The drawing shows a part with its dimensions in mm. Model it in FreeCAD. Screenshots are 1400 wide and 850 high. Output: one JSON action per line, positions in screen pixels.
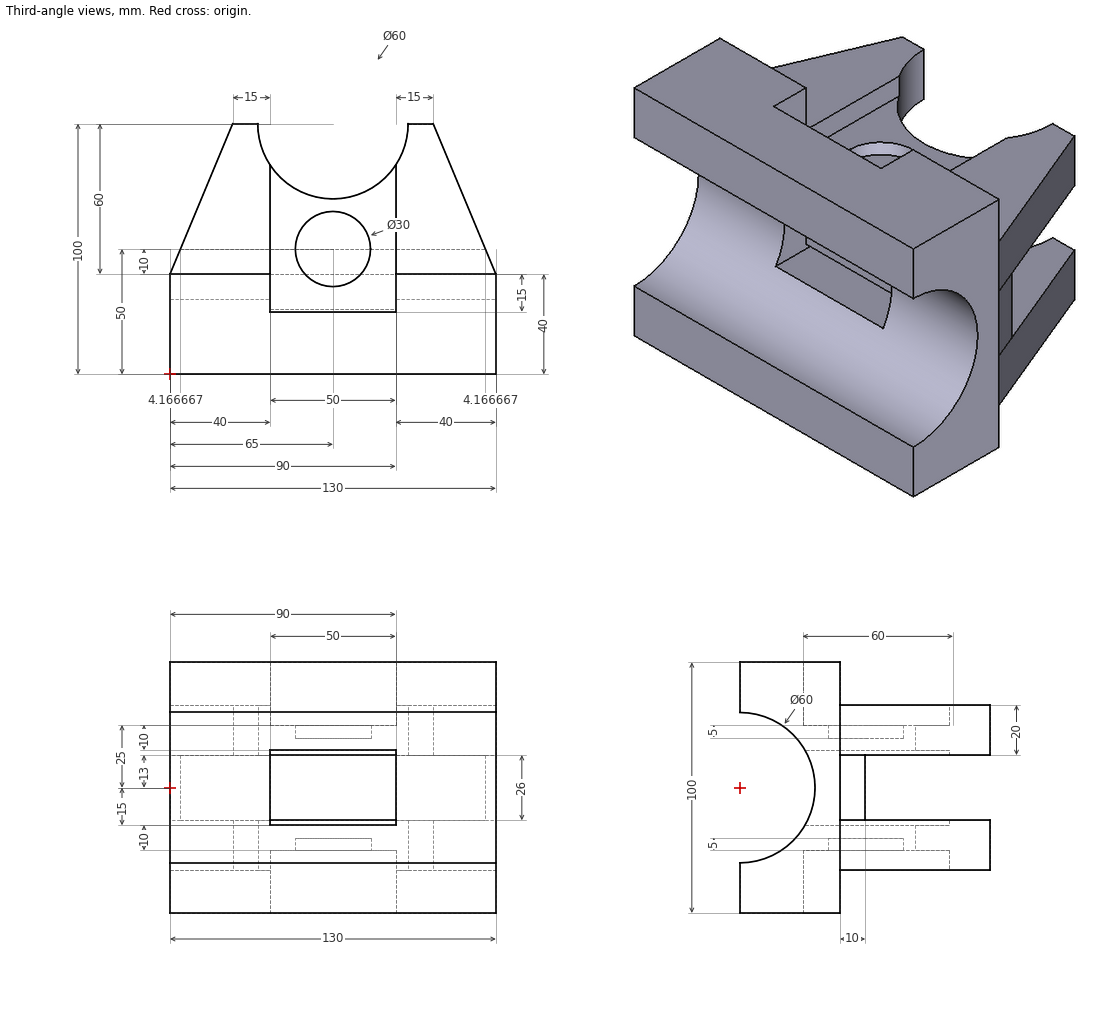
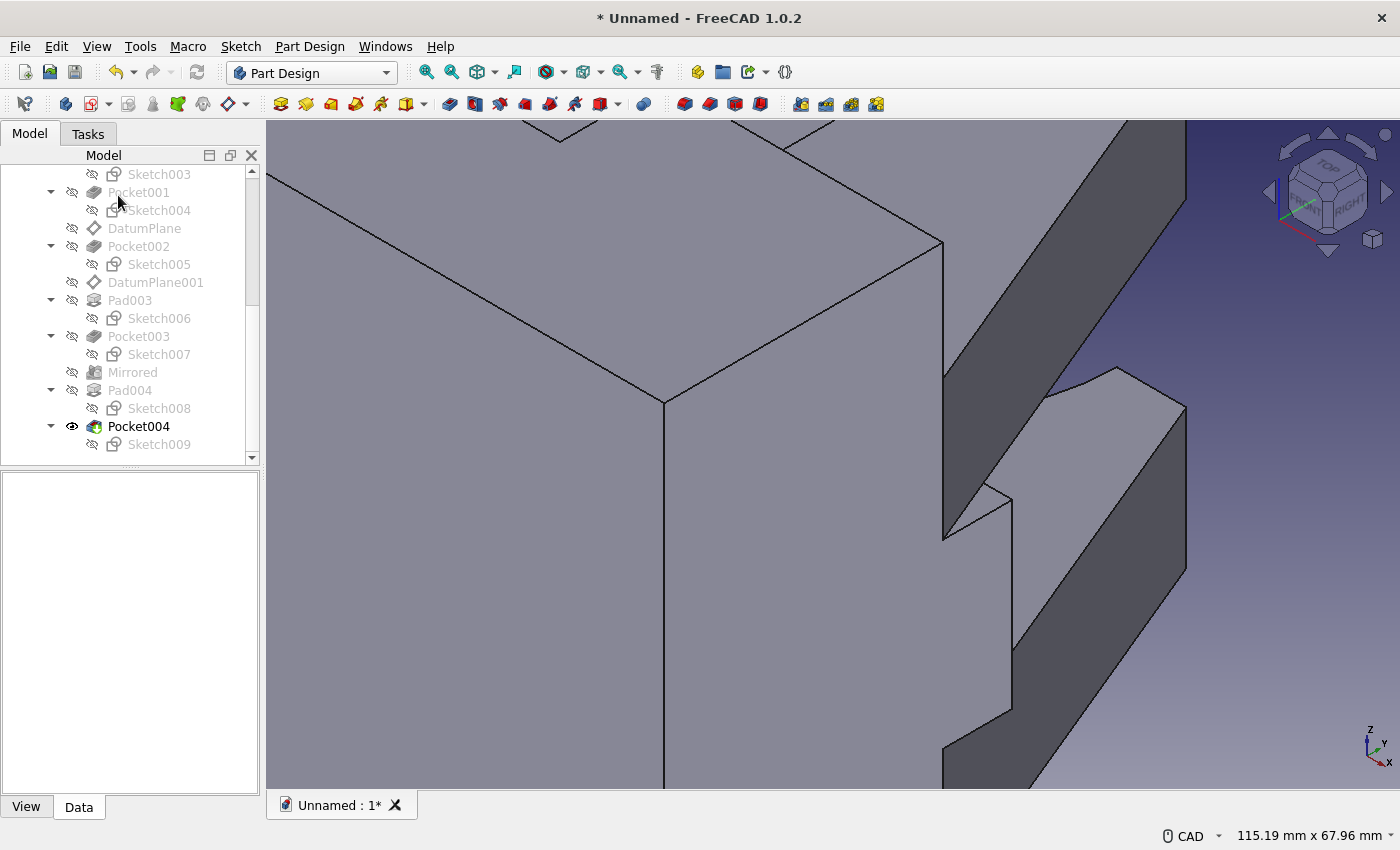
{"action": "left_click", "coordinate": [427, 72]}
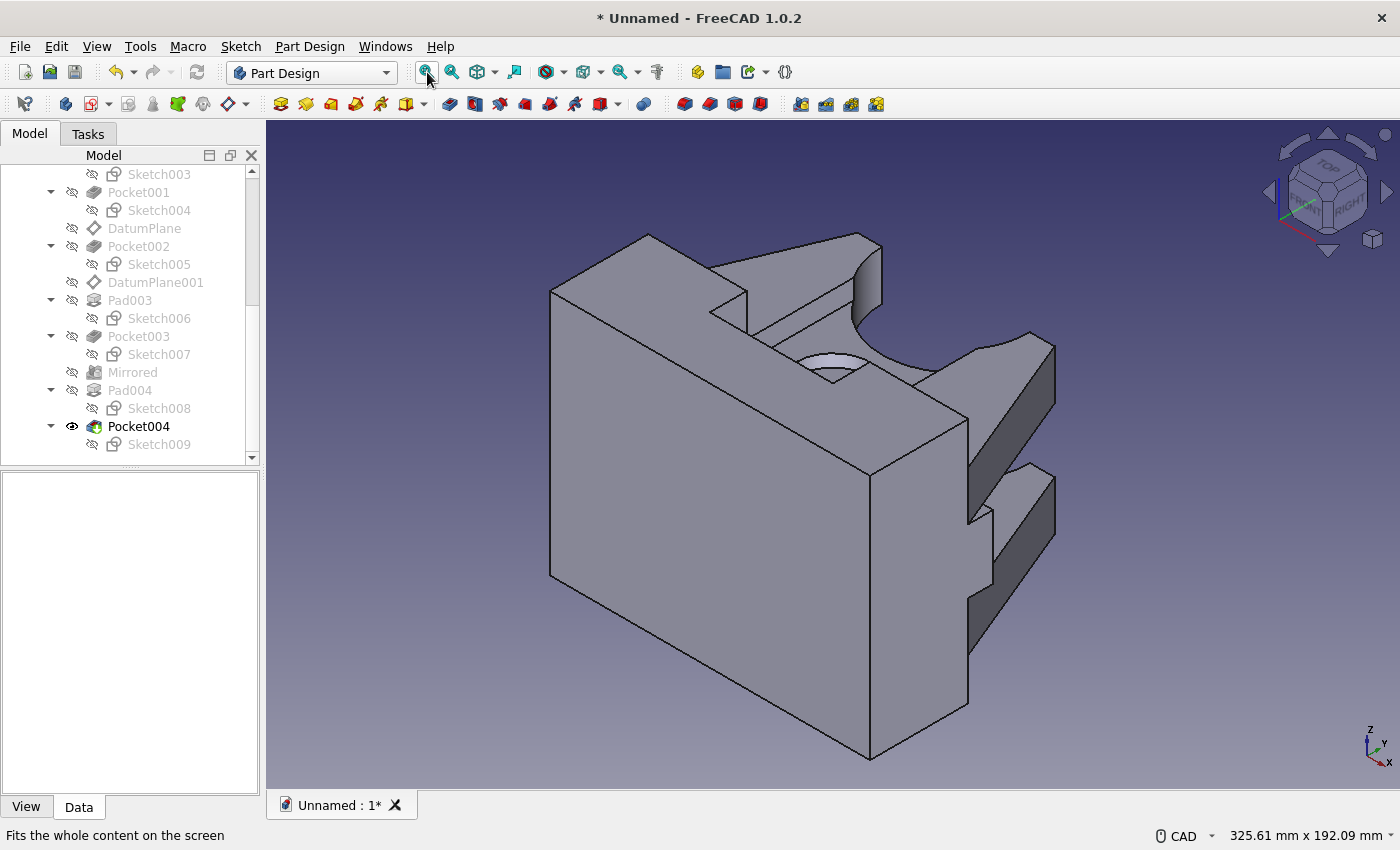
{"action": "scroll", "coordinate": [984, 510], "scroll_direction": "up", "scroll_amount": 5}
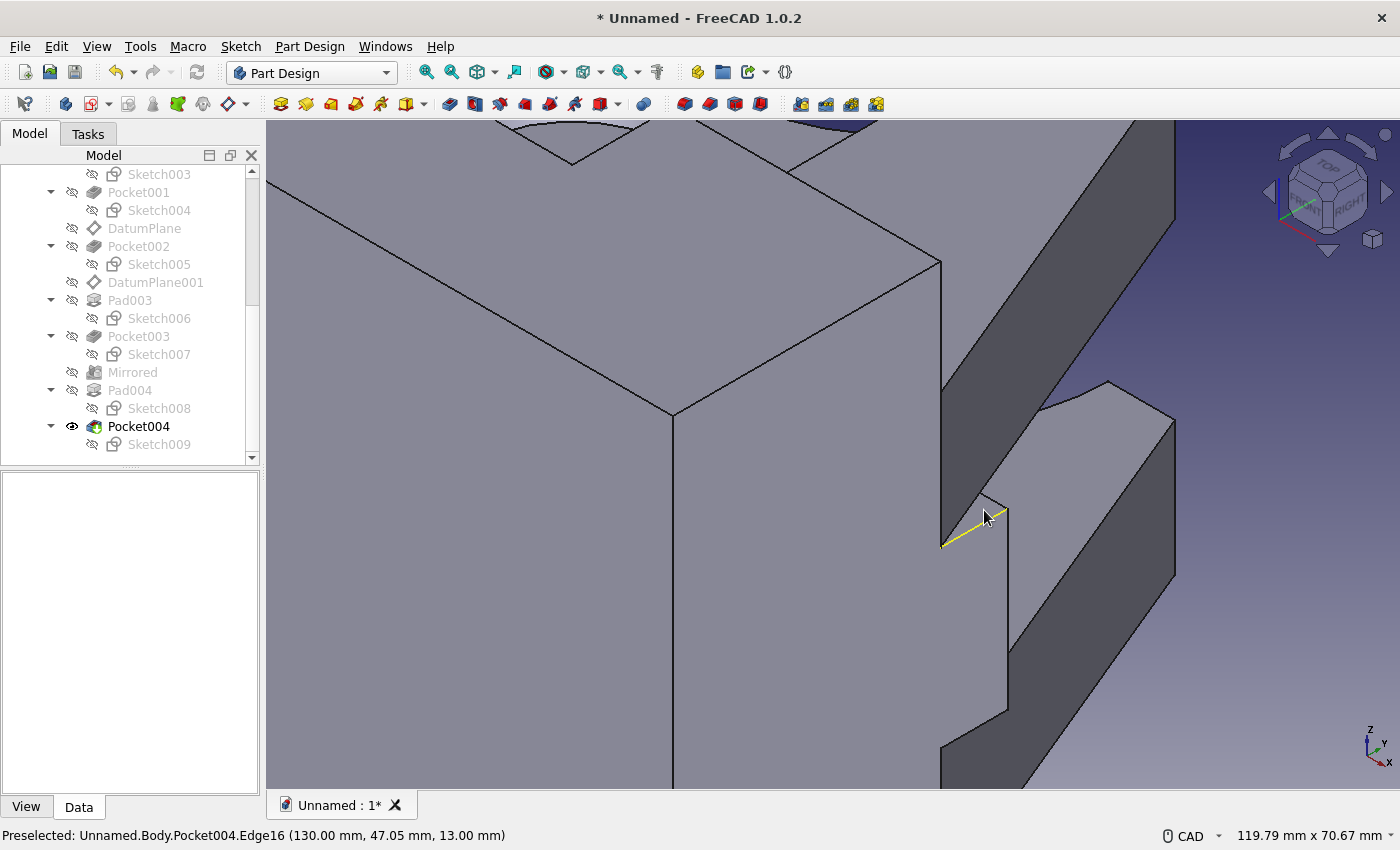
{"action": "left_click", "coordinate": [983, 510]}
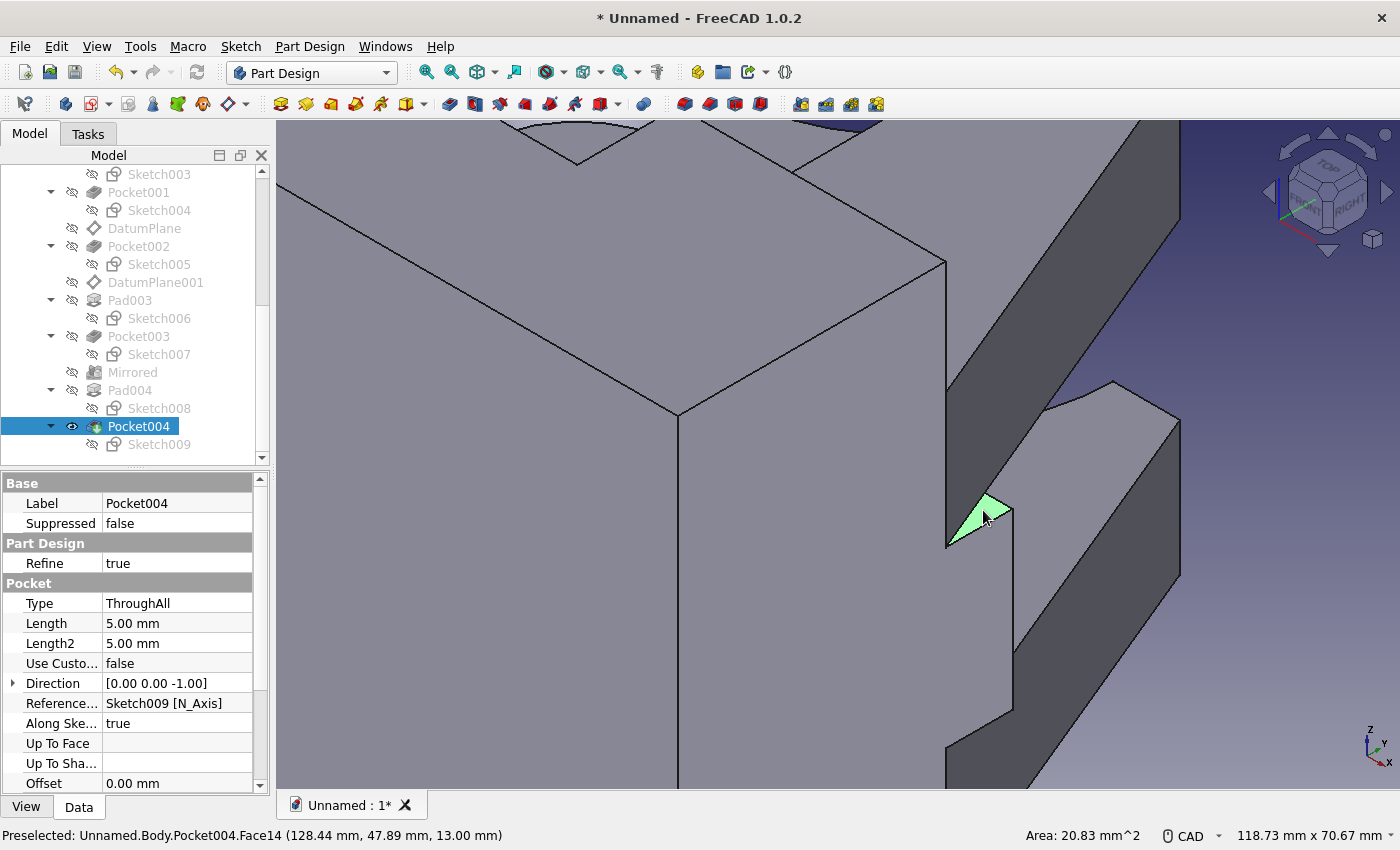
{"action": "left_click", "coordinate": [90, 104]}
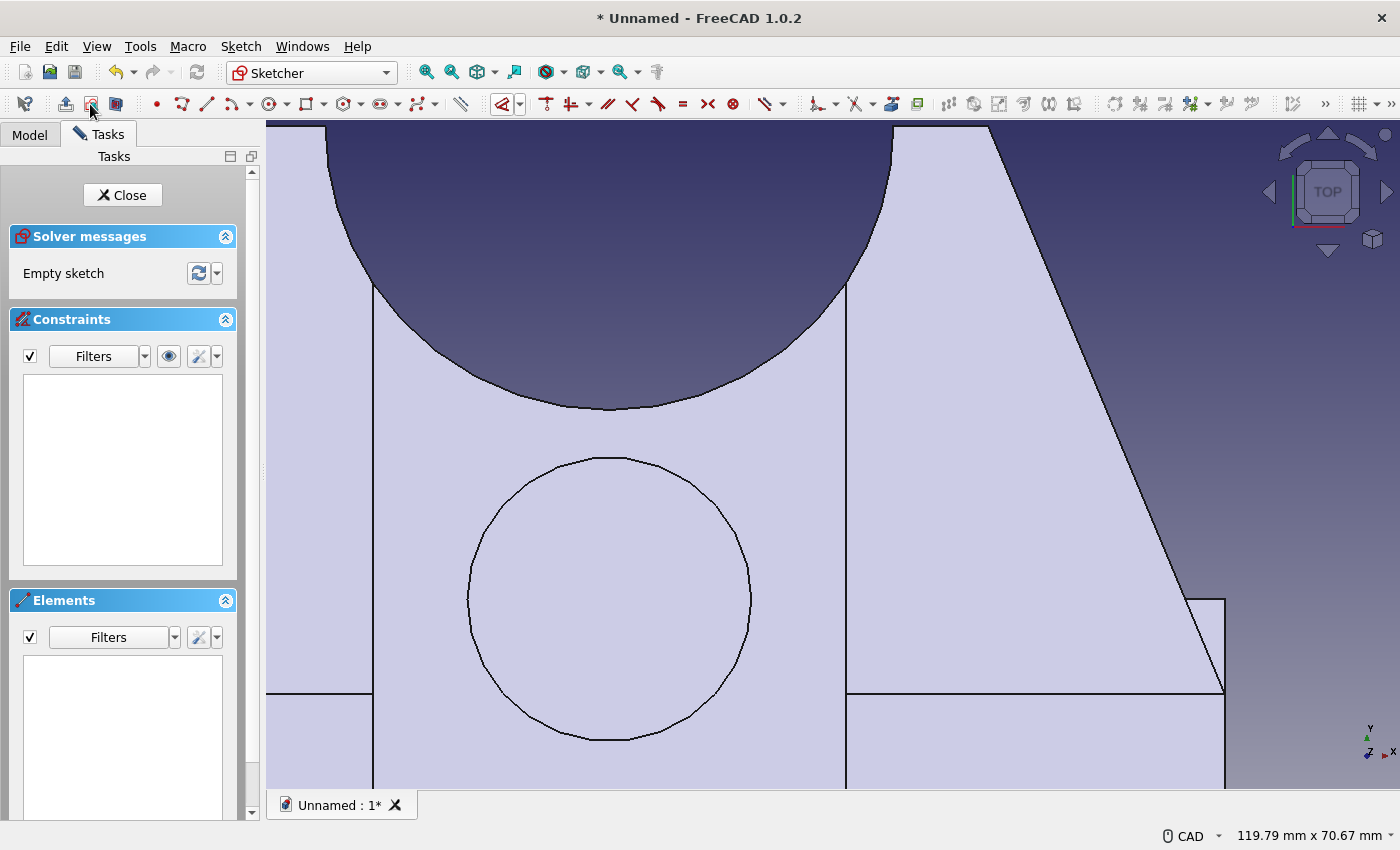
{"action": "scroll", "coordinate": [1235, 695], "scroll_direction": "up", "scroll_amount": 8}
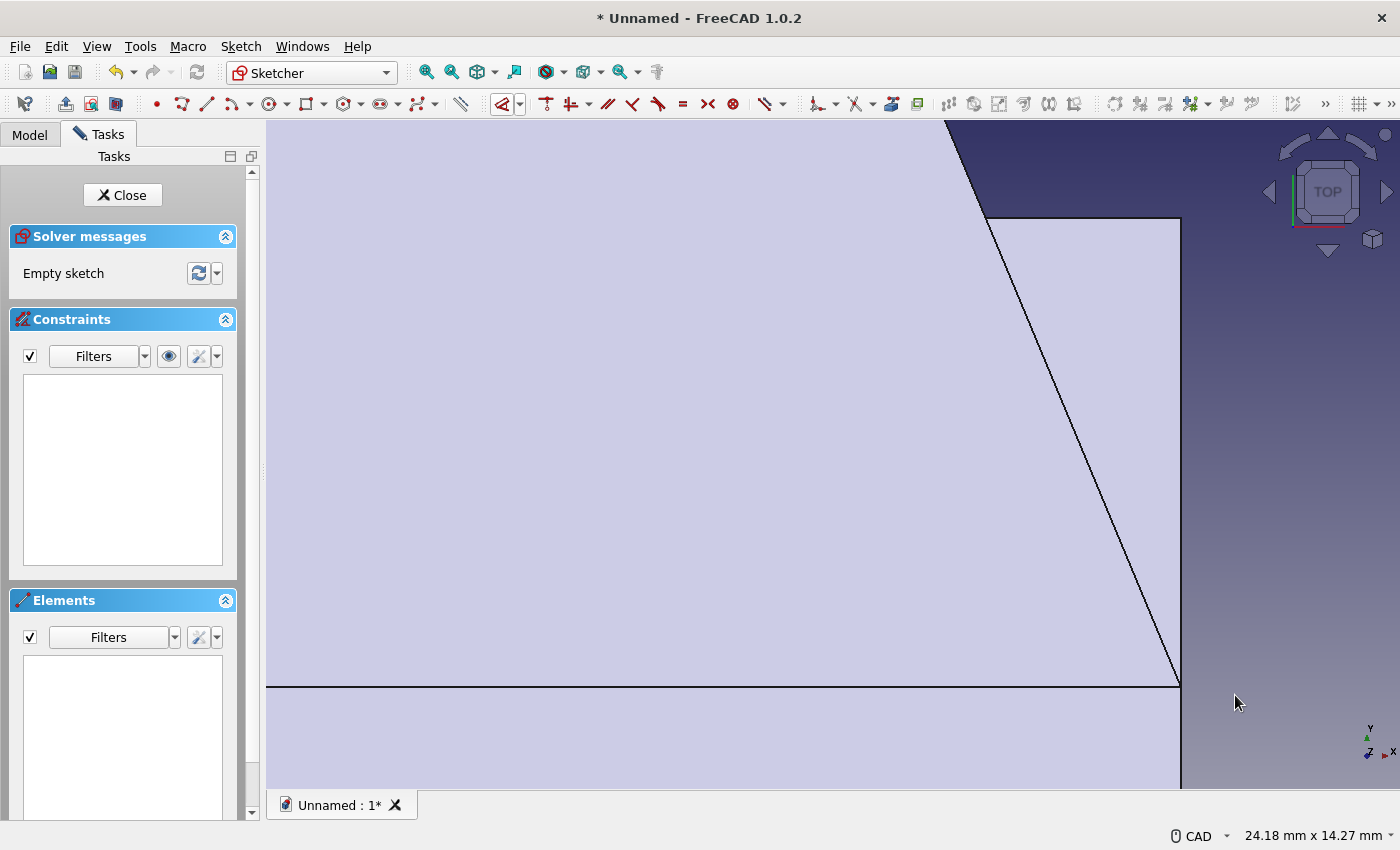
{"action": "left_click", "coordinate": [182, 104]}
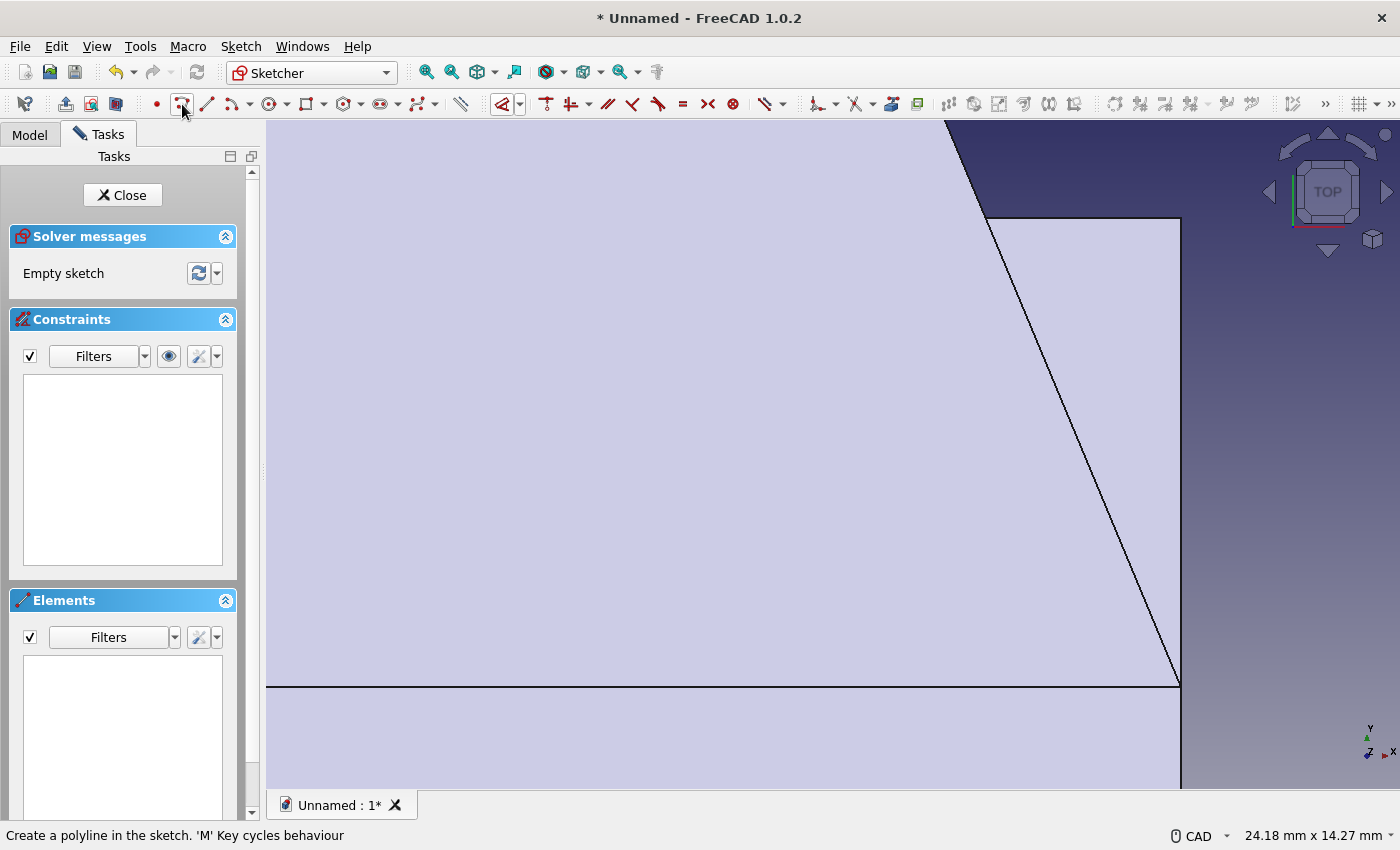
{"action": "left_click", "coordinate": [986, 218]}
{"action": "left_click", "coordinate": [1181, 687]}
{"action": "left_click", "coordinate": [1181, 218]}
{"action": "left_click", "coordinate": [986, 219]}
{"action": "key", "text": "Escape"}
{"action": "key", "text": "Escape"}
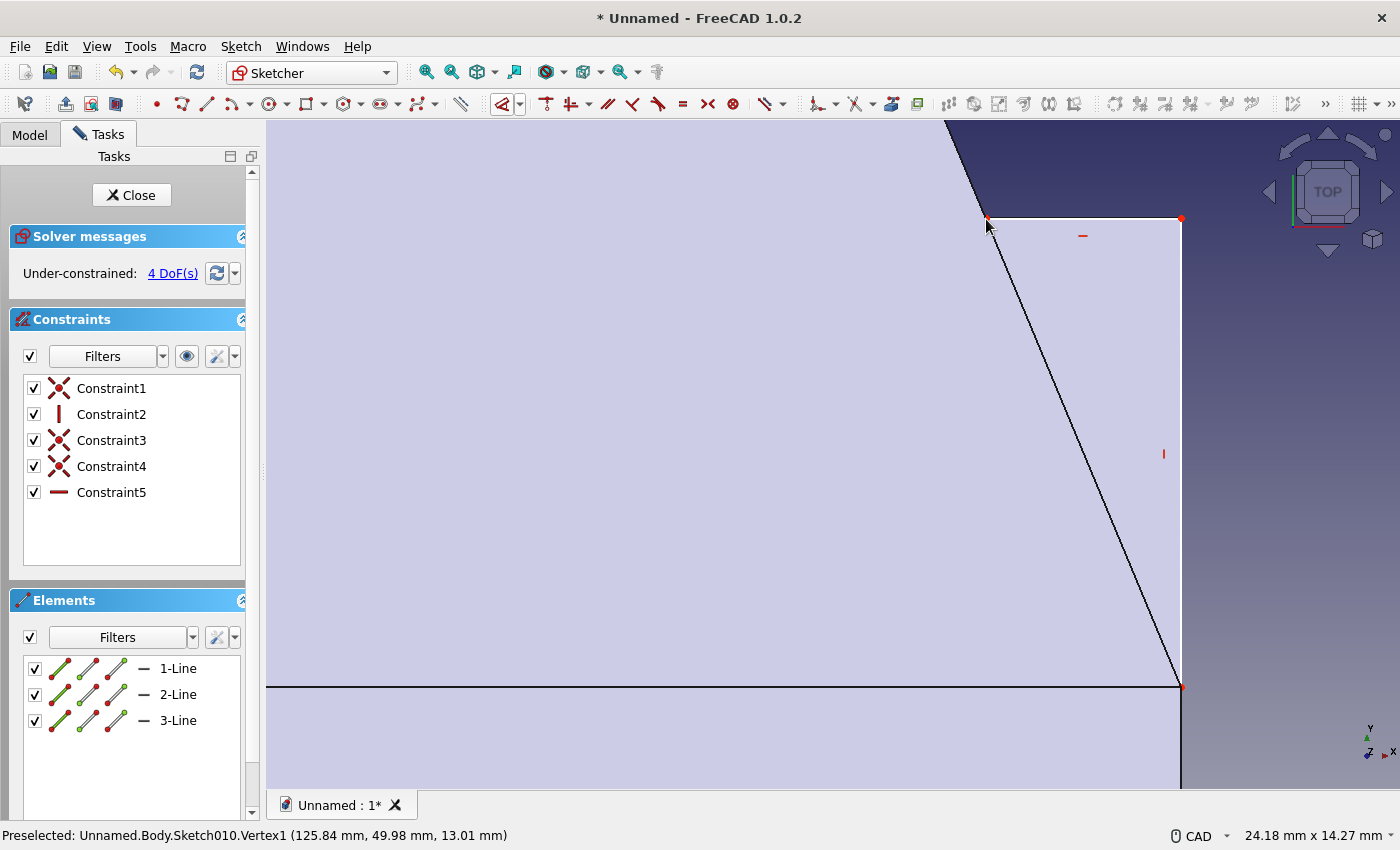
{"action": "left_click", "coordinate": [1181, 547]}